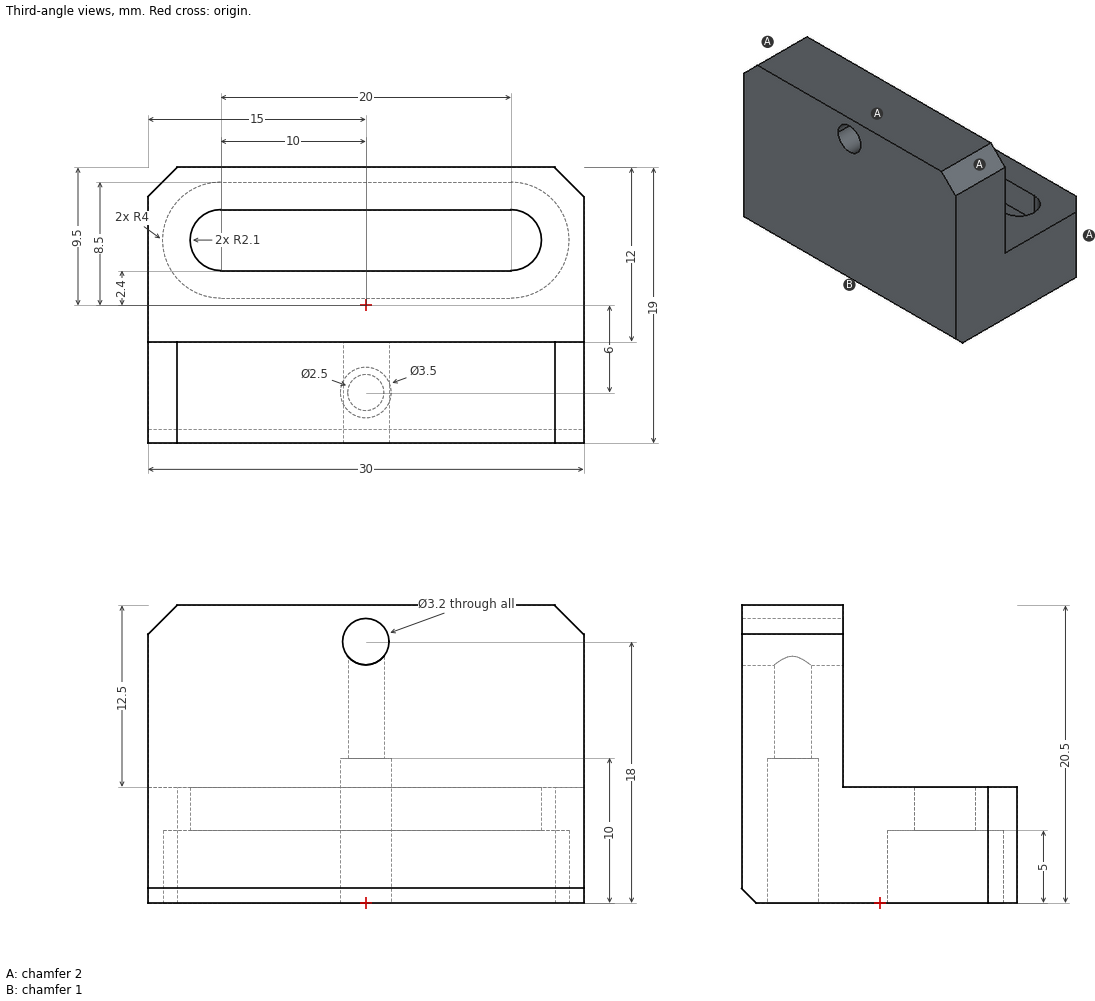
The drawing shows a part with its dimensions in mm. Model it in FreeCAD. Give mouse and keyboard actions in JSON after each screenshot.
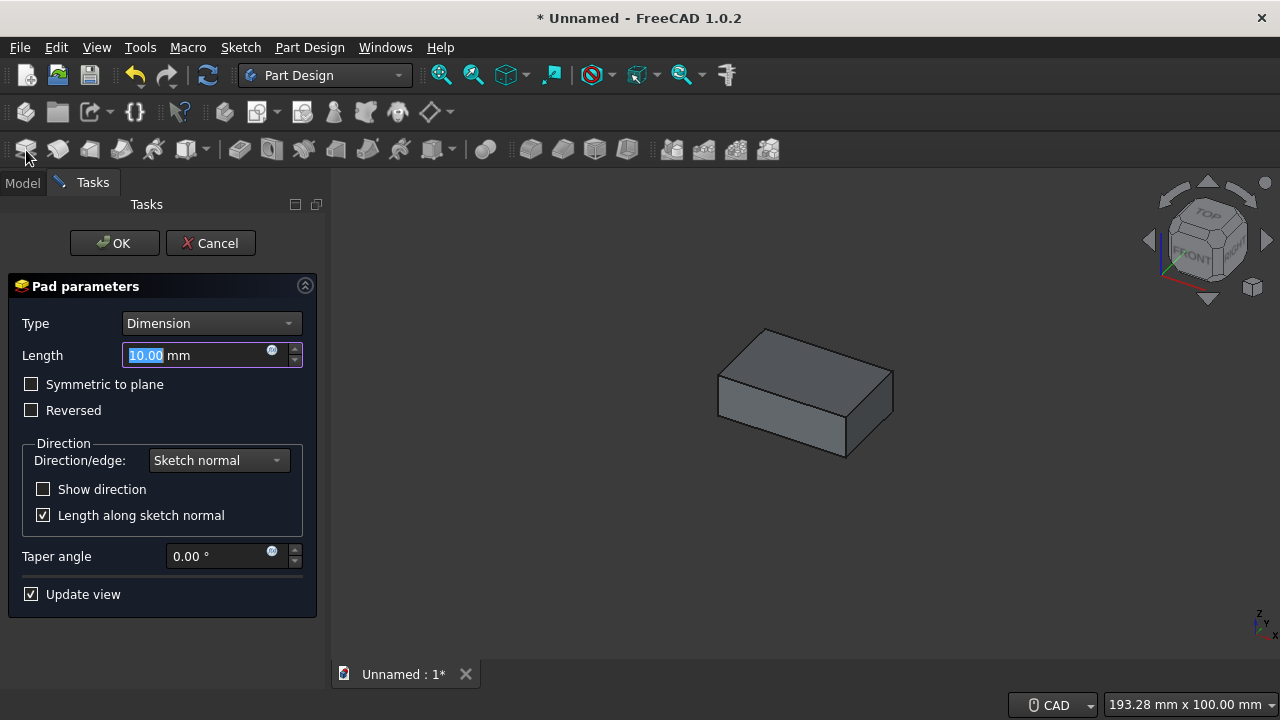
{"action": "type", "text": "20.5"}
{"action": "key", "text": "Tab"}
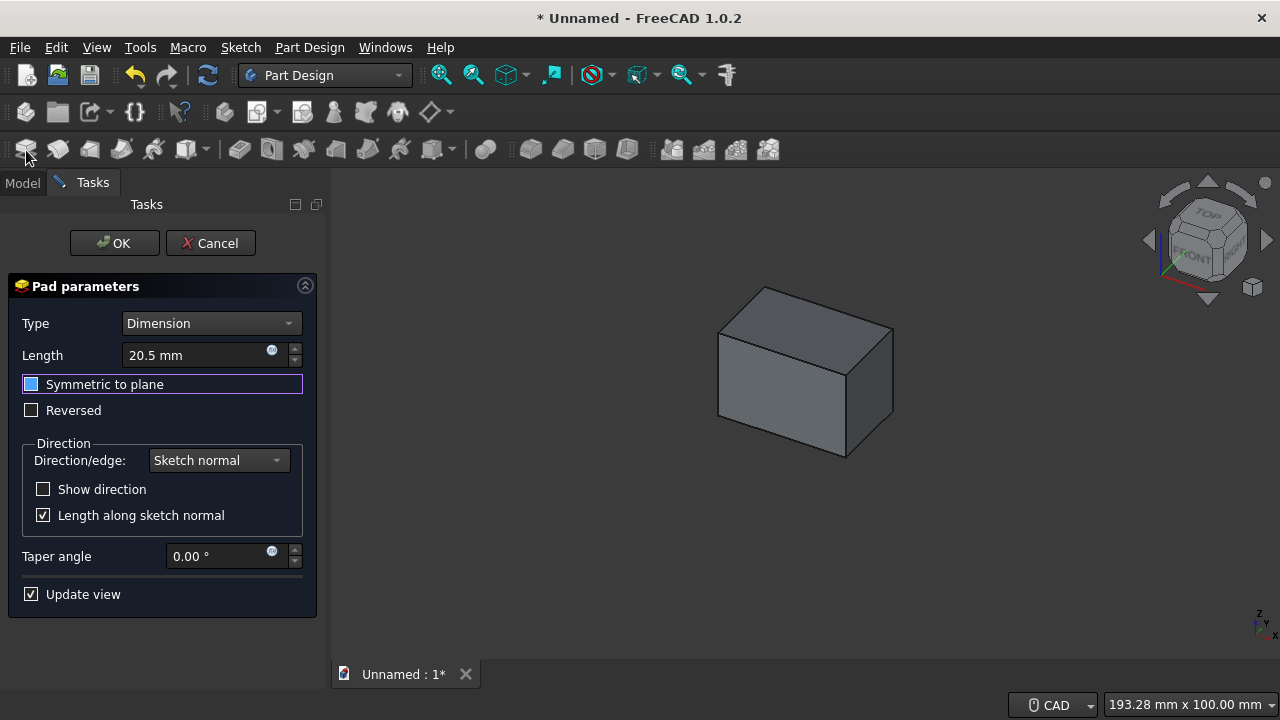
{"action": "left_click", "coordinate": [115, 243]}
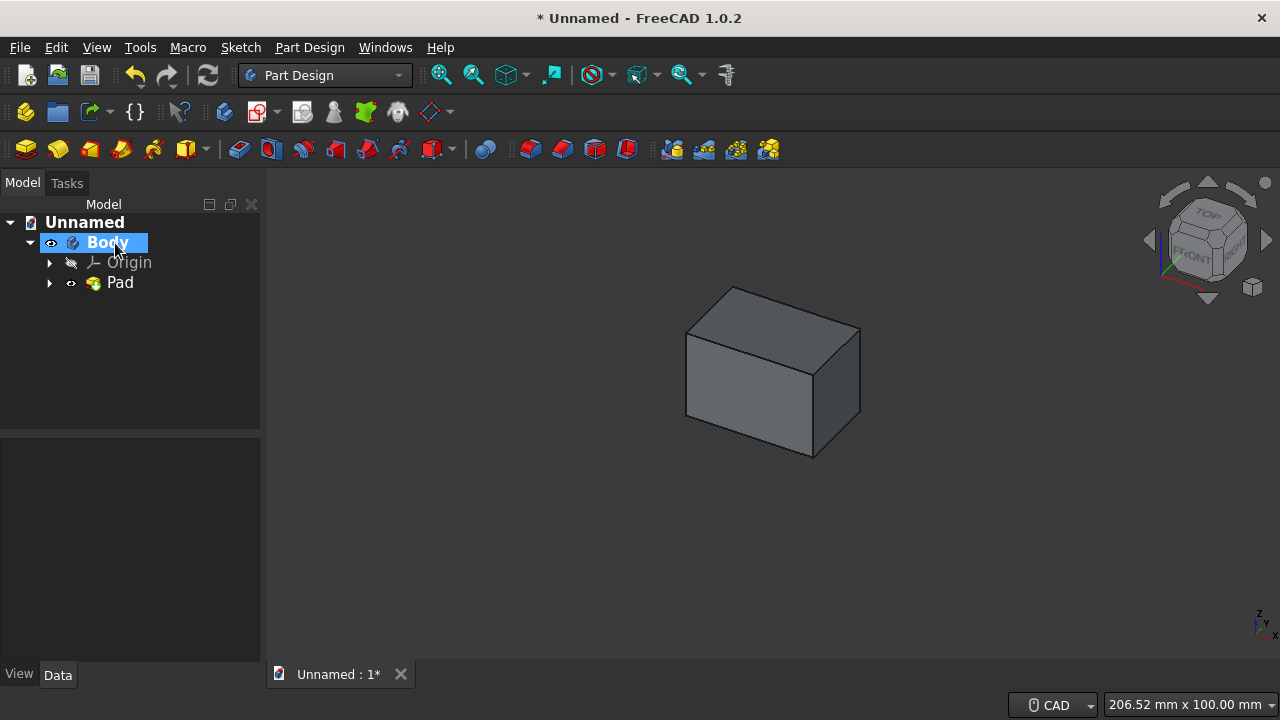
{"action": "key", "text": "v f"}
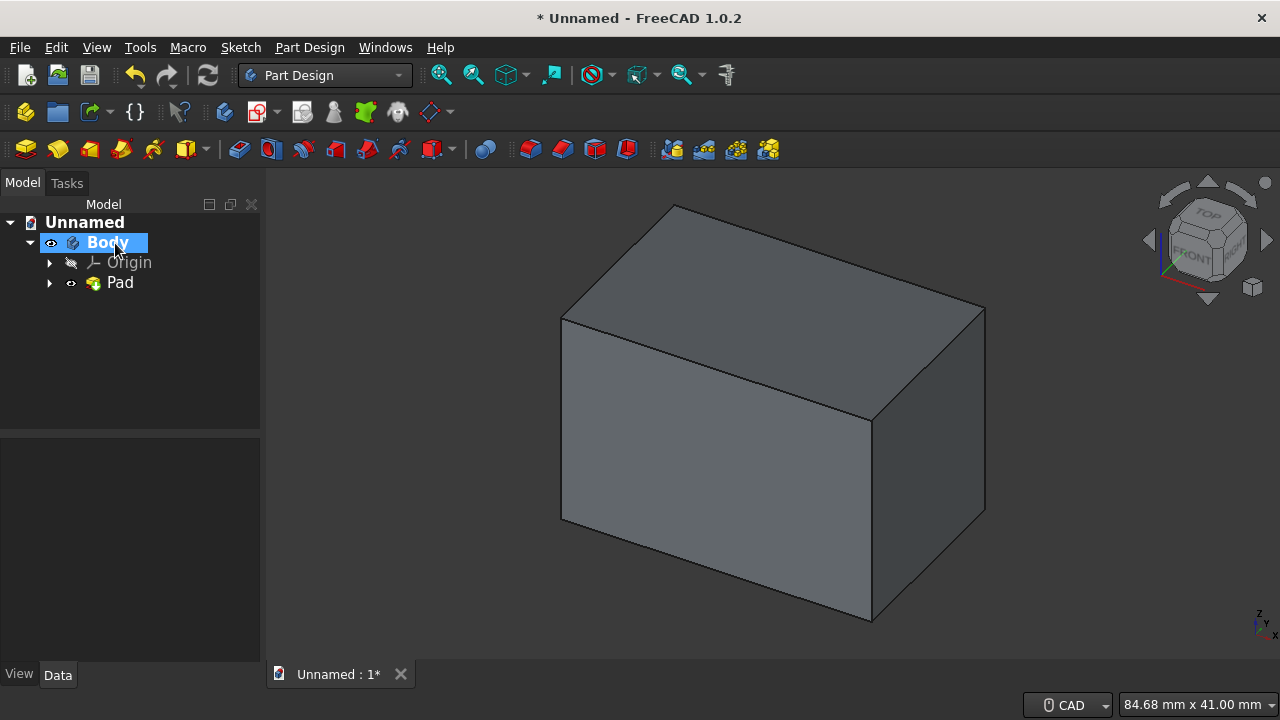
{"action": "left_click", "coordinate": [817, 327]}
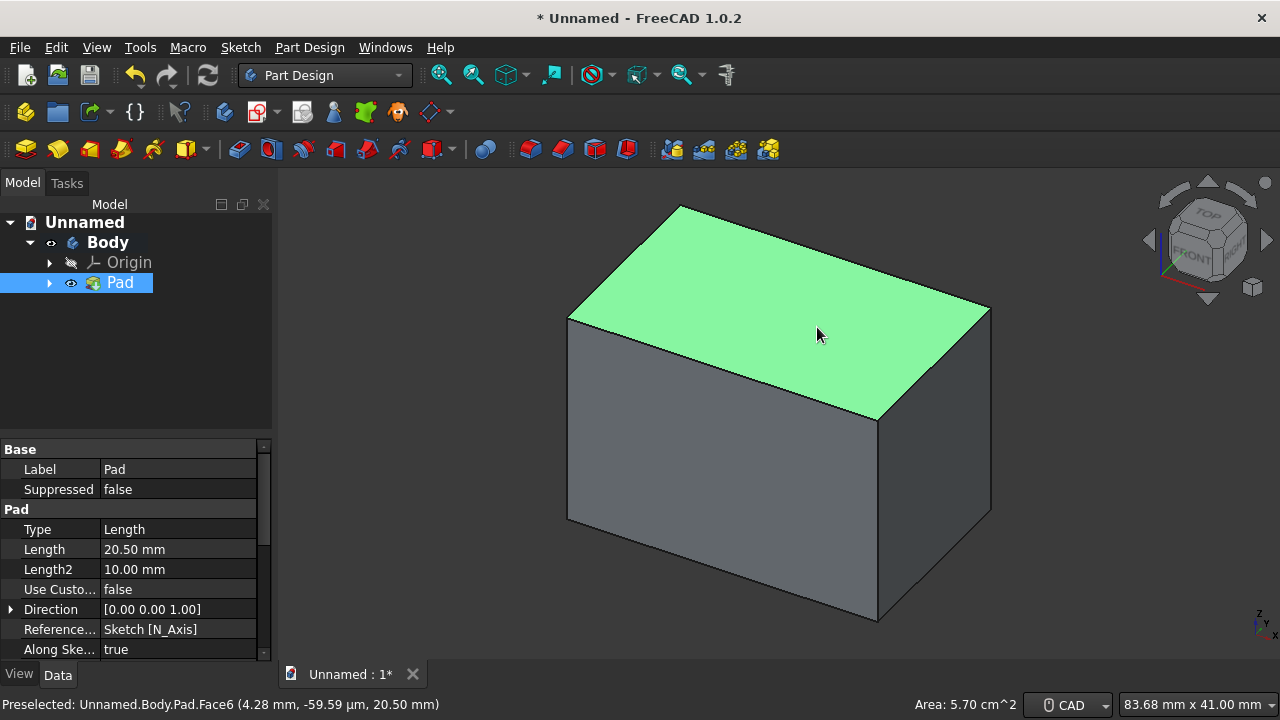
{"action": "left_click", "coordinate": [258, 112]}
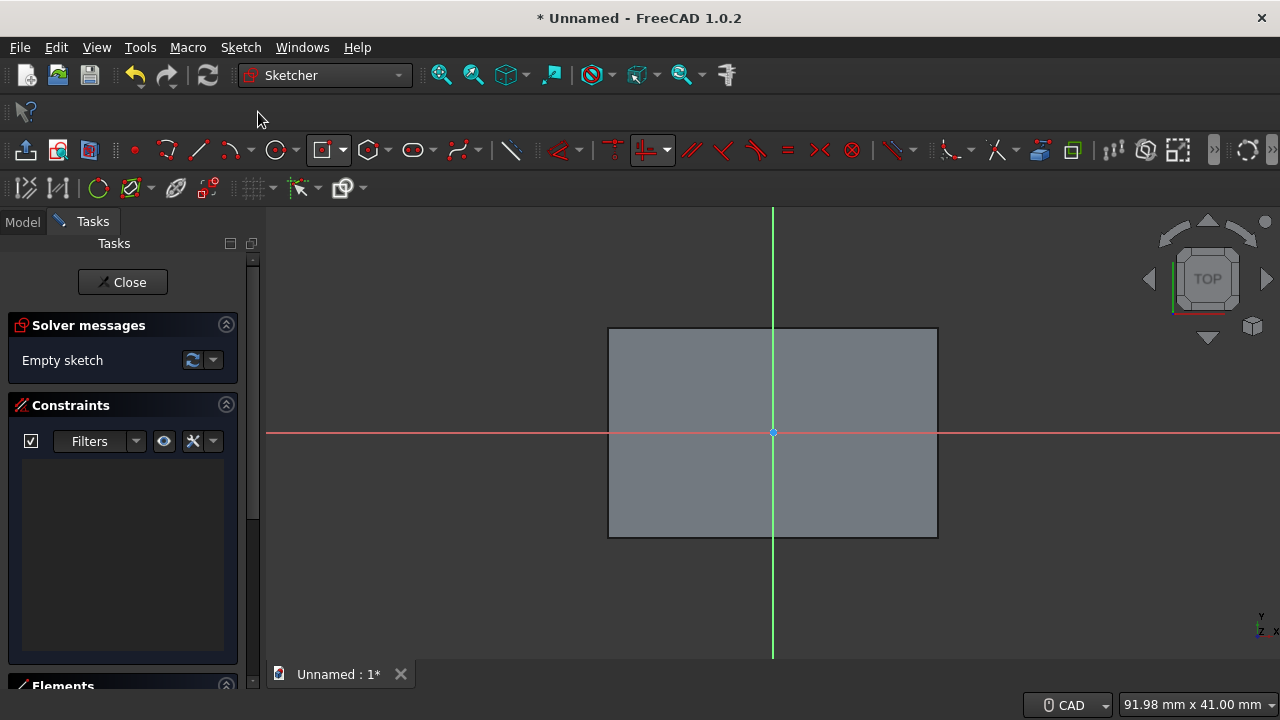
{"action": "scroll", "coordinate": [856, 347], "scroll_direction": "up", "scroll_amount": 3}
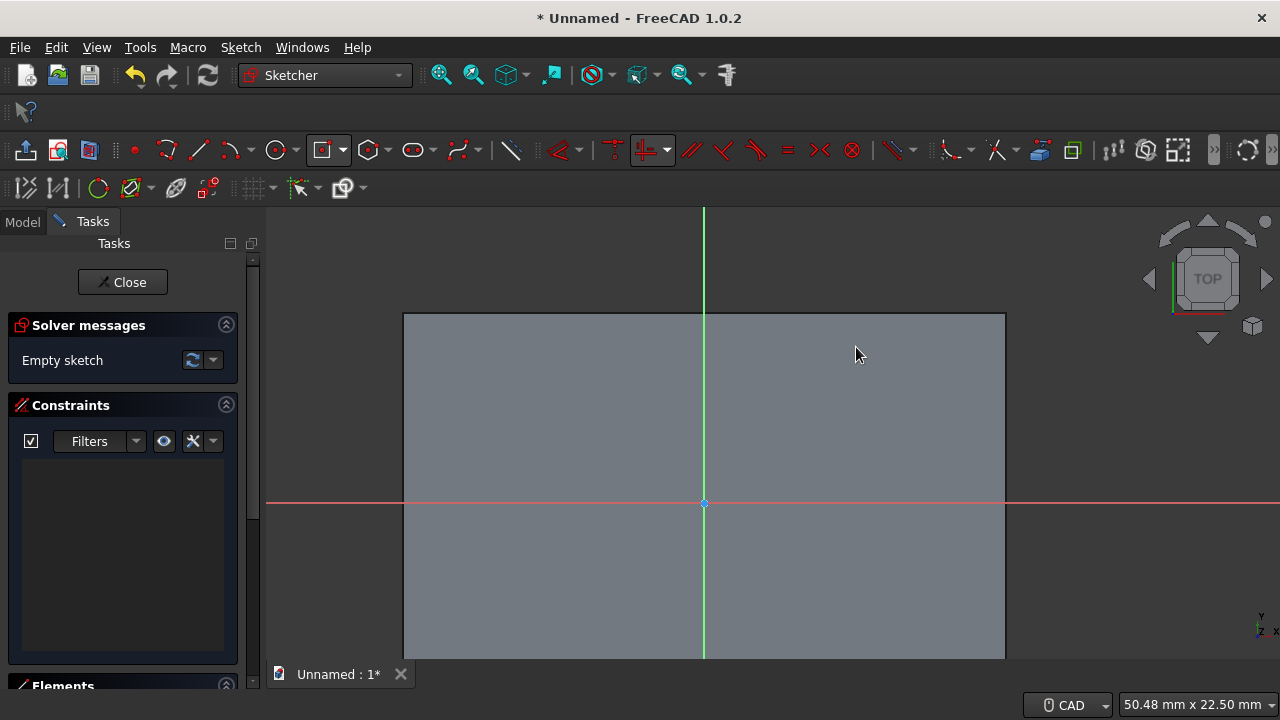
{"action": "key", "text": "g r"}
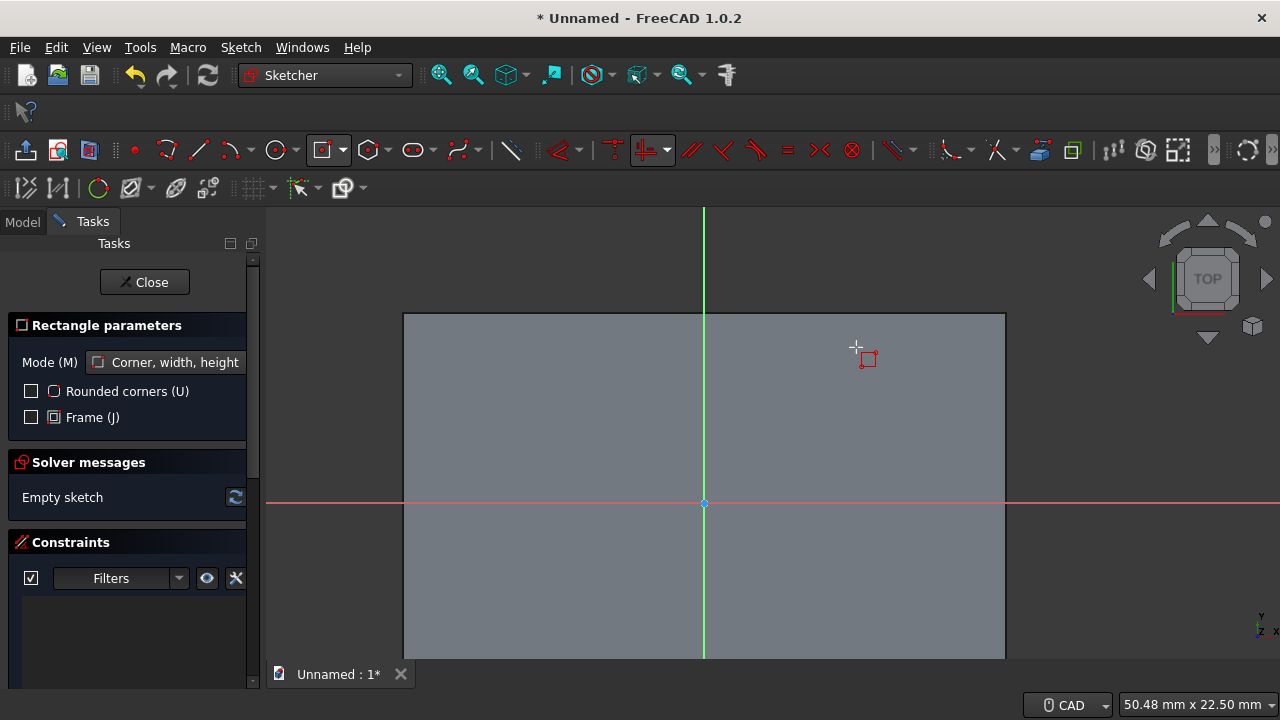
{"action": "left_click", "coordinate": [403, 313]}
{"action": "mouse_move", "coordinate": [1006, 554]}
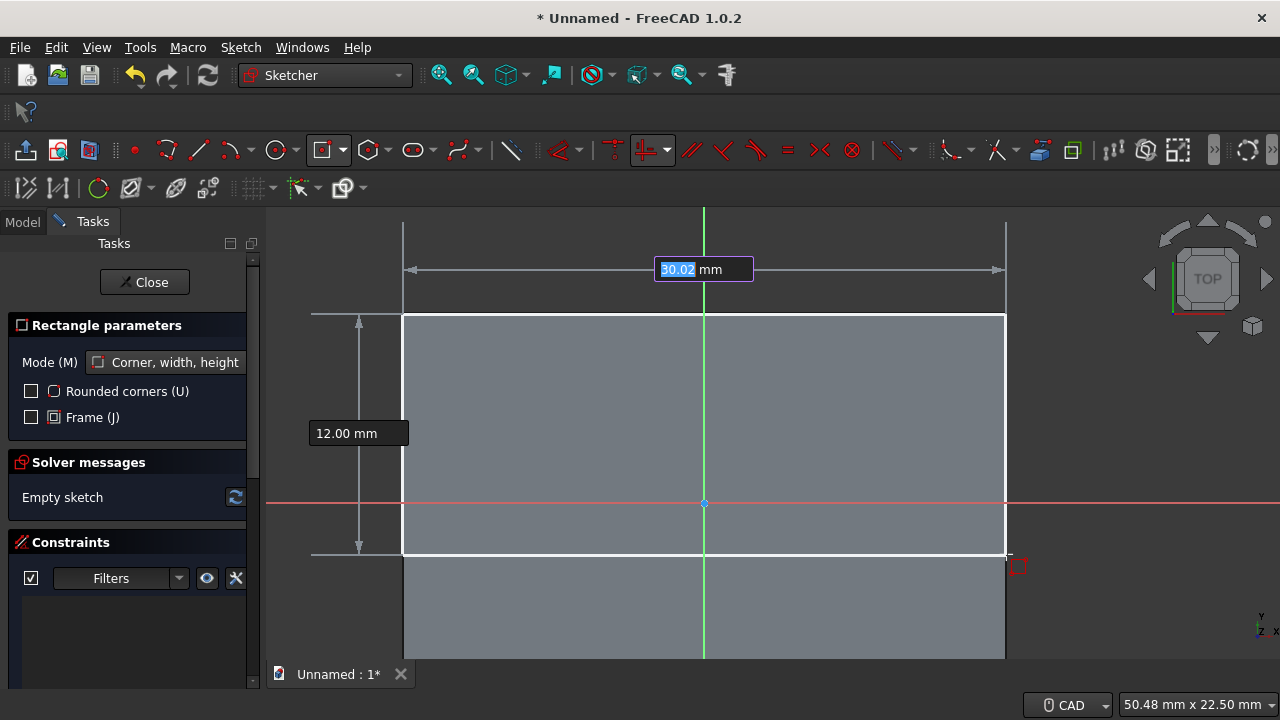
{"action": "type", "text": "30"}
{"action": "key", "text": "Tab"}
{"action": "type", "text": "12"}
{"action": "key", "text": "Return"}
{"action": "key", "text": "Escape"}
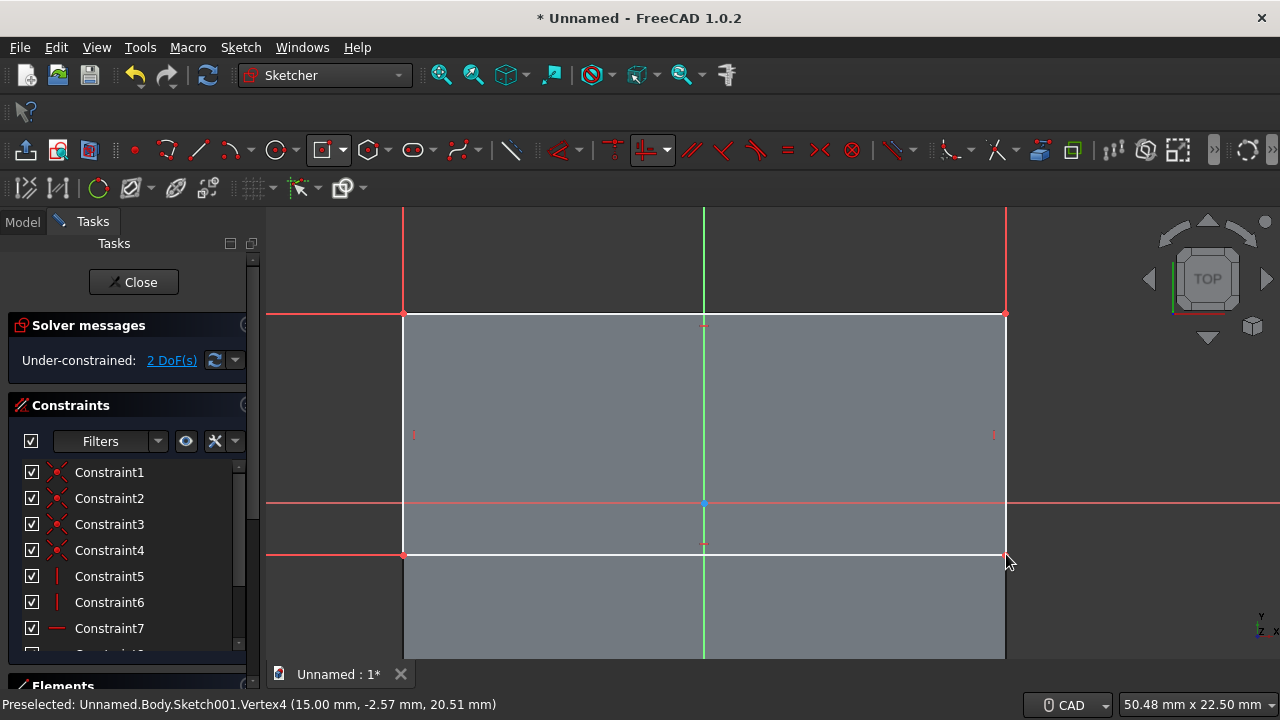
{"action": "left_click", "coordinate": [403, 314]}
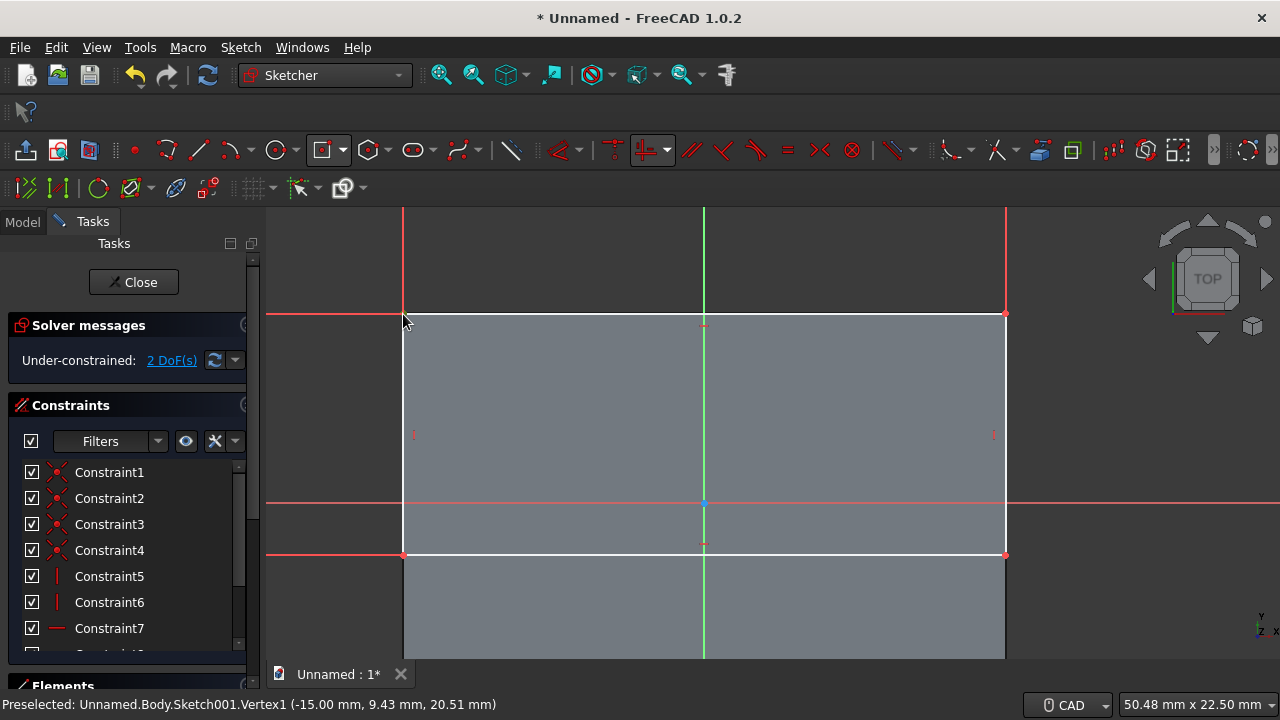
{"action": "key", "text": "l"}